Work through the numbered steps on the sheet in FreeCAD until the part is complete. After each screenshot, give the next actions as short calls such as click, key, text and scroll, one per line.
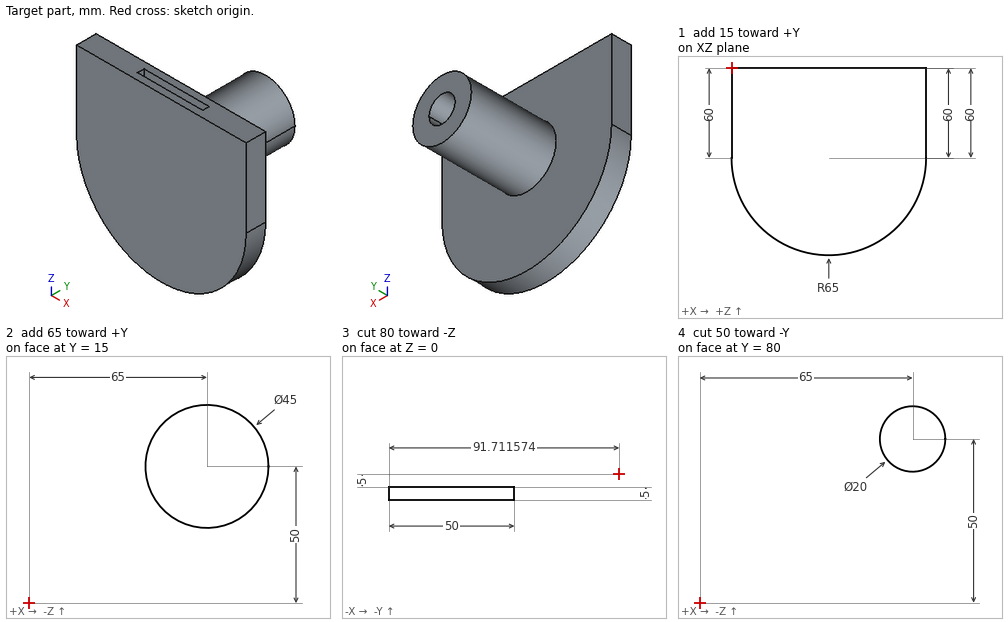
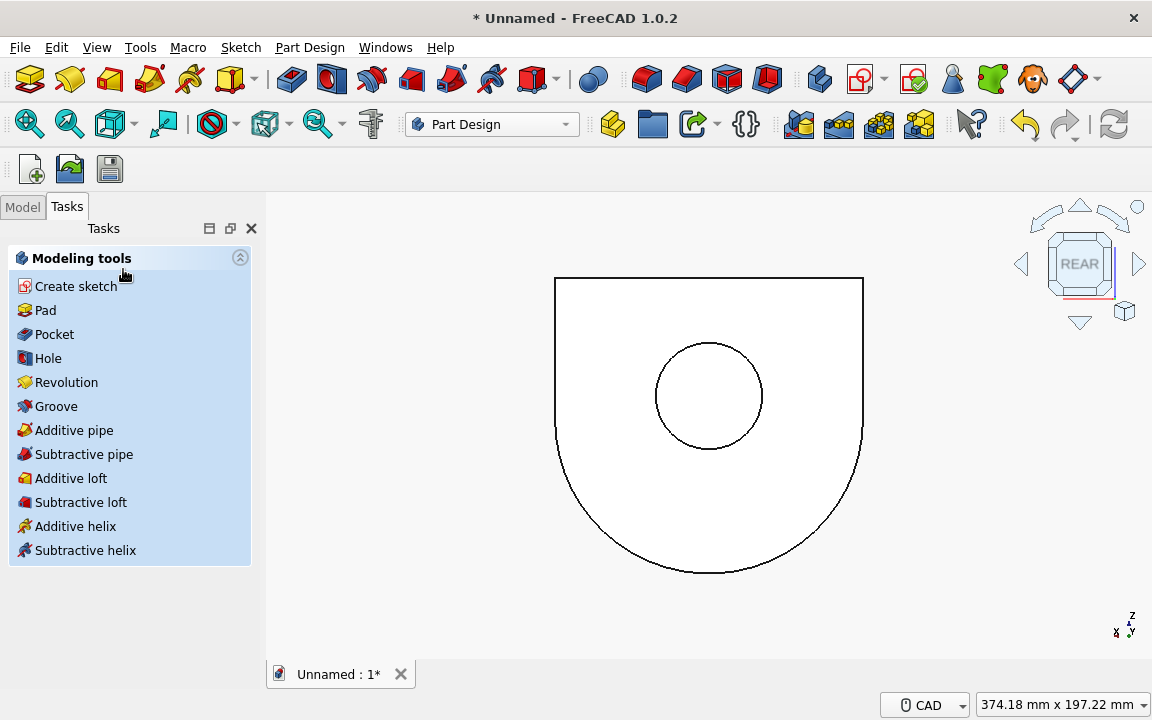
click(292, 80)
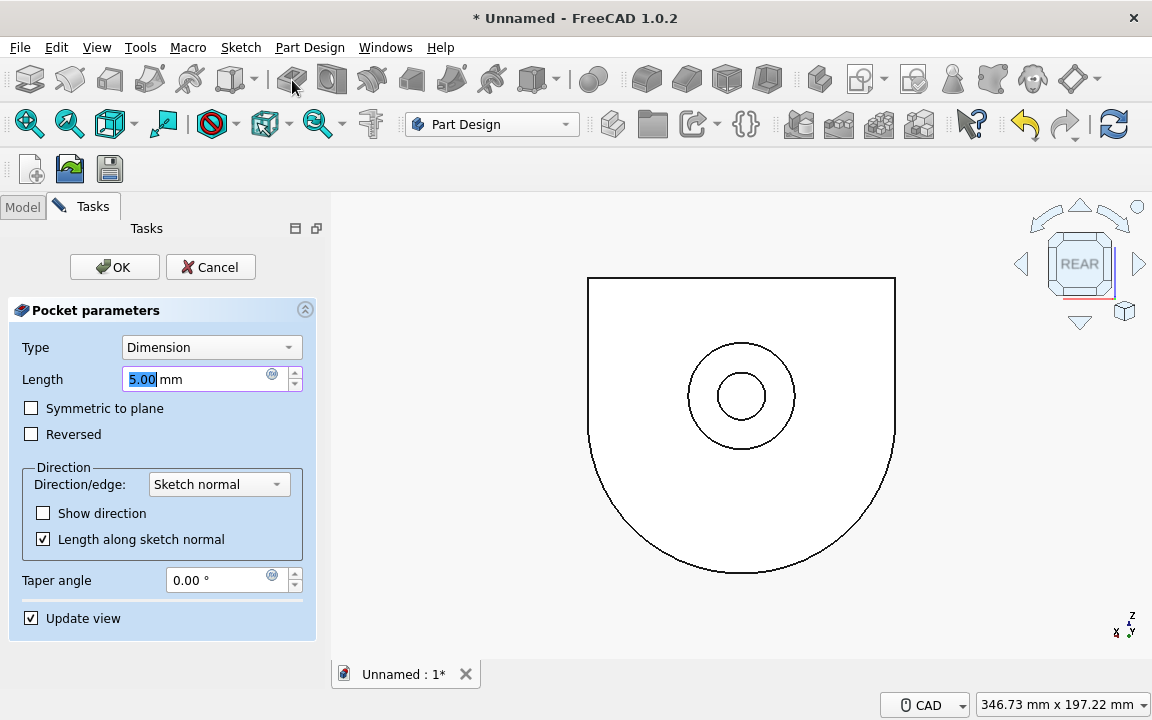
text(50)
key(Tab)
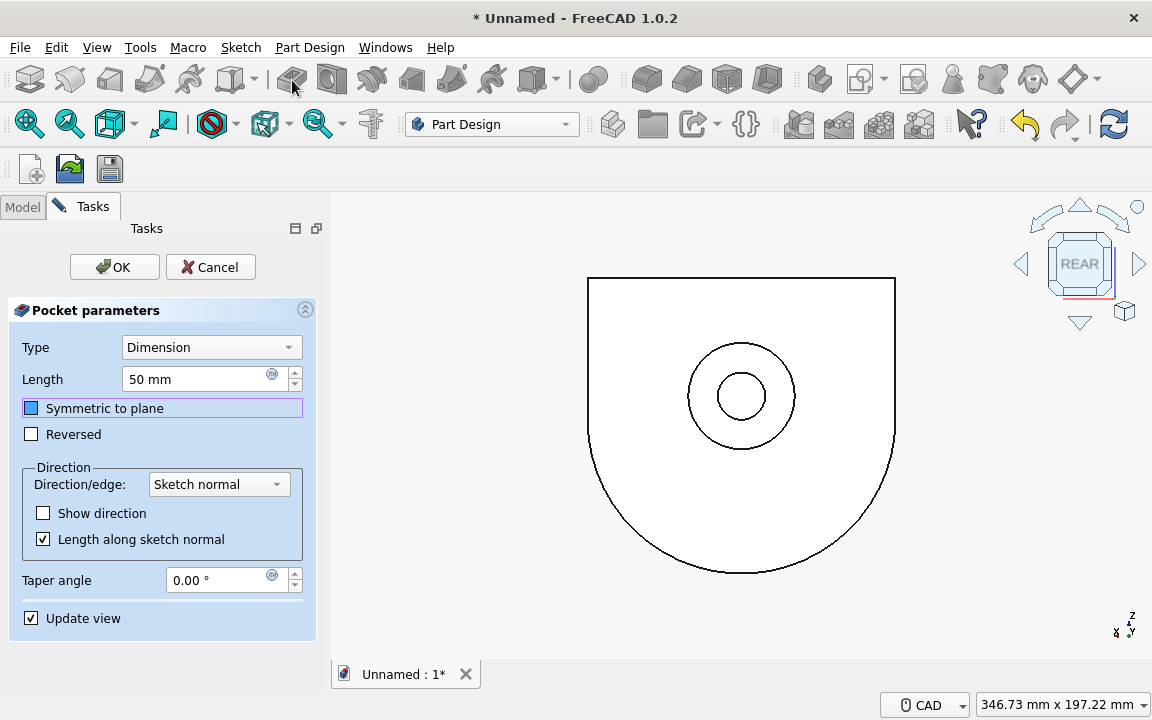
click(115, 267)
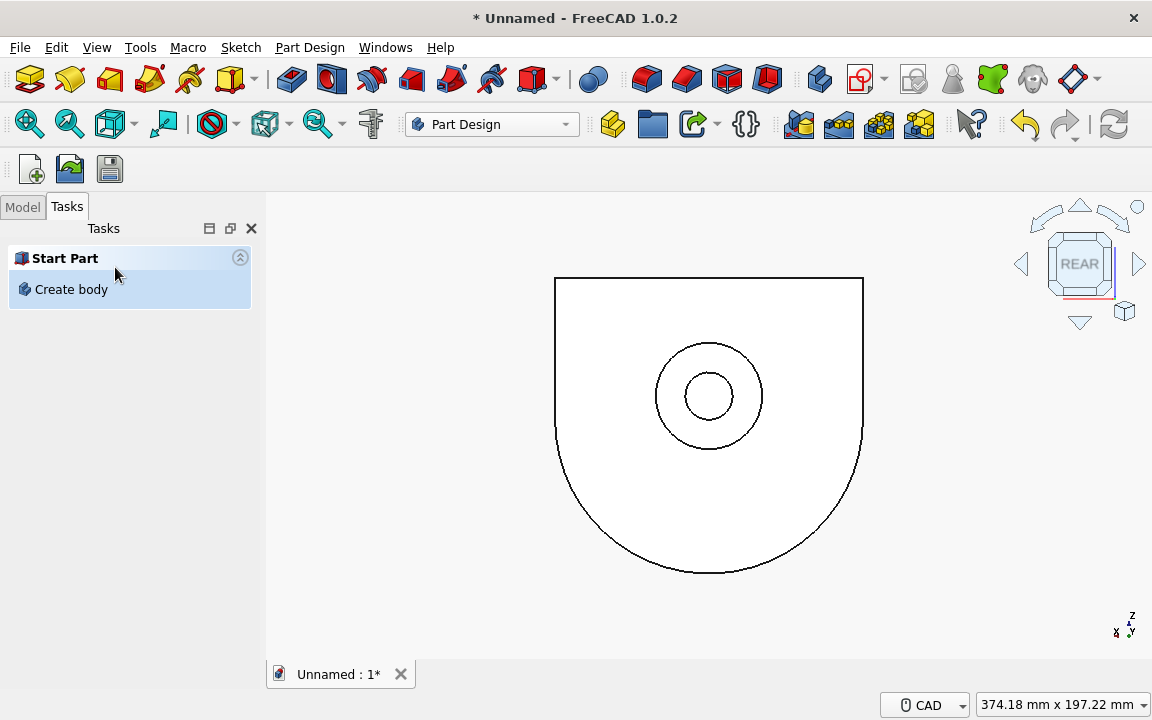
key(0)